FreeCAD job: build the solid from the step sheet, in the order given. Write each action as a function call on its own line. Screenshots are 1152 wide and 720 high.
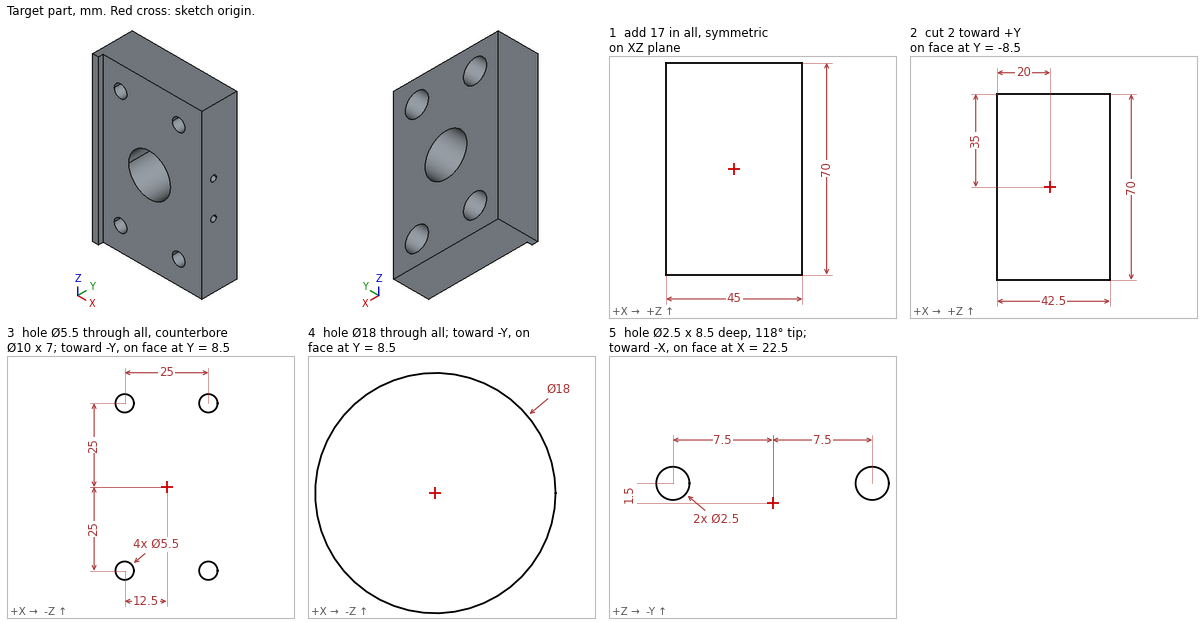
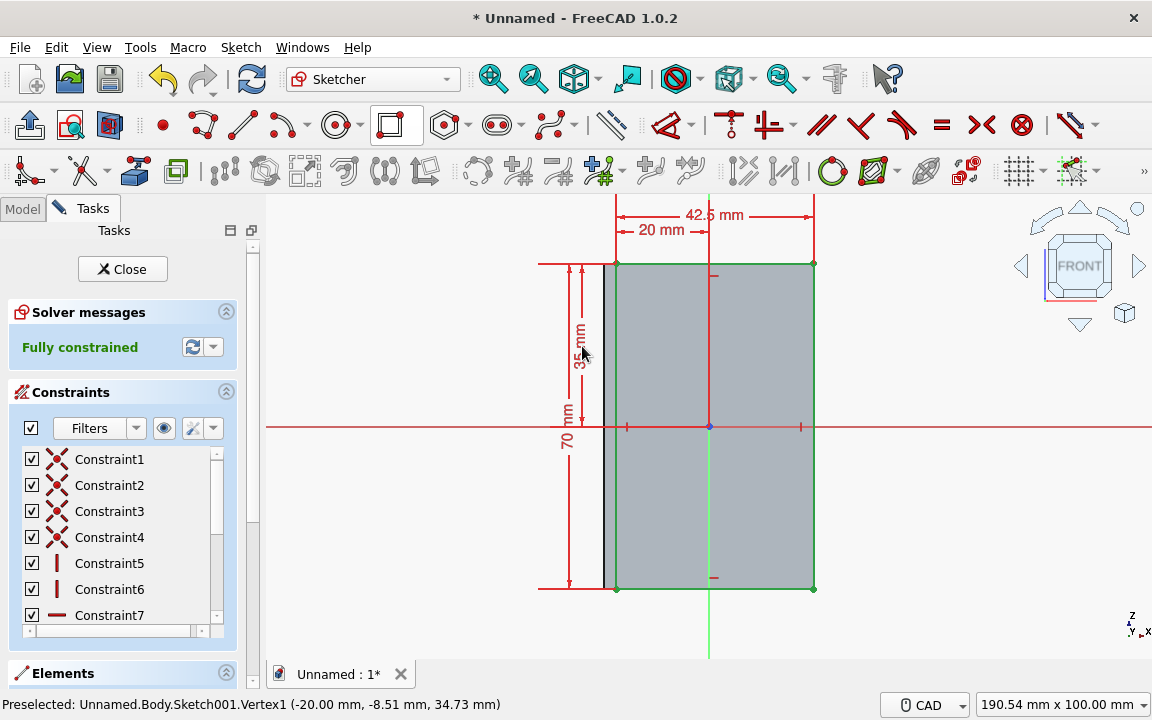
click(123, 269)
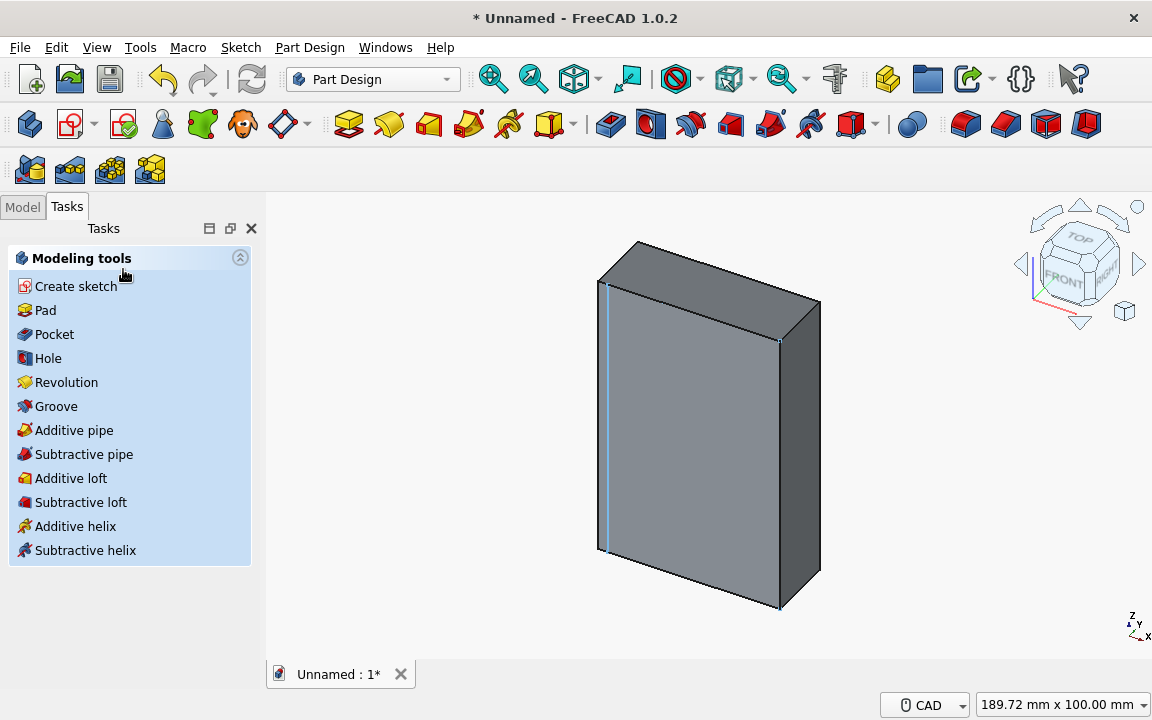
click(612, 124)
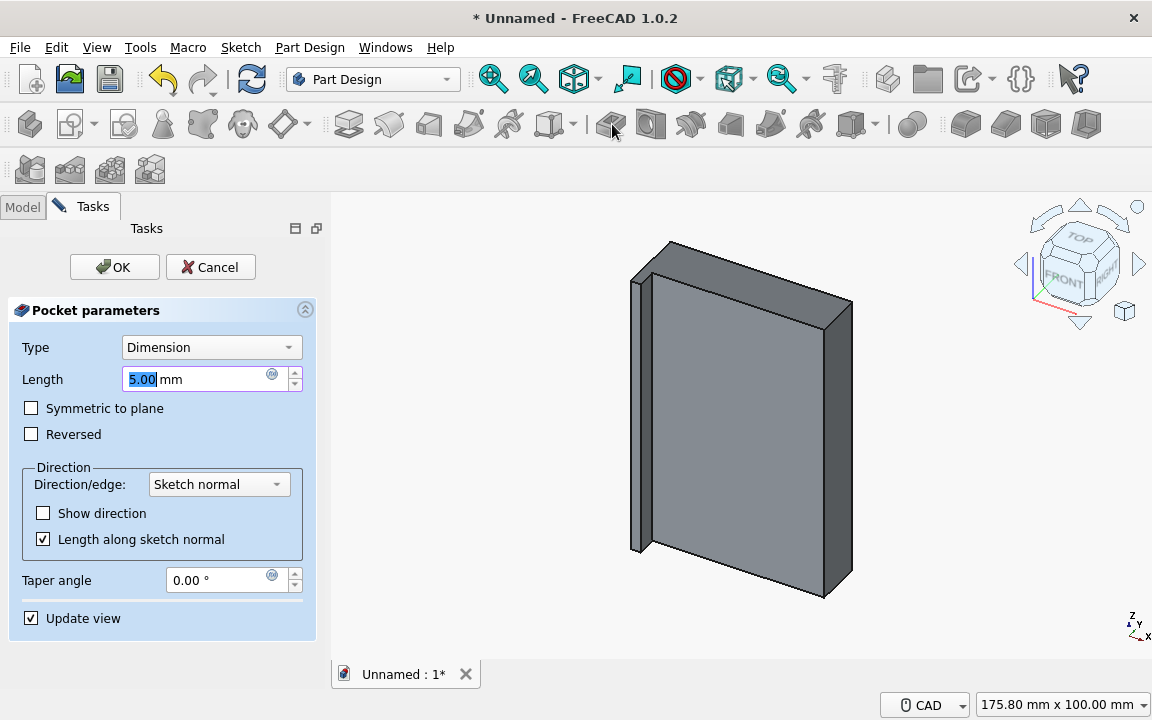
text(2)
key(Tab)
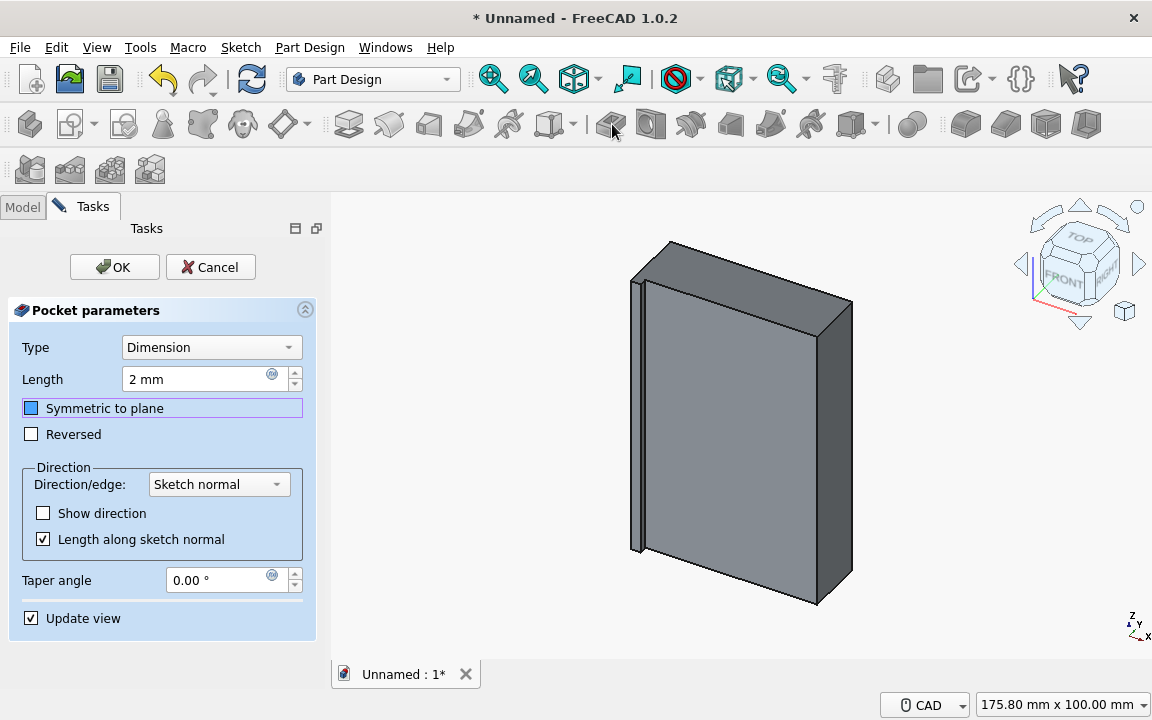
click(115, 267)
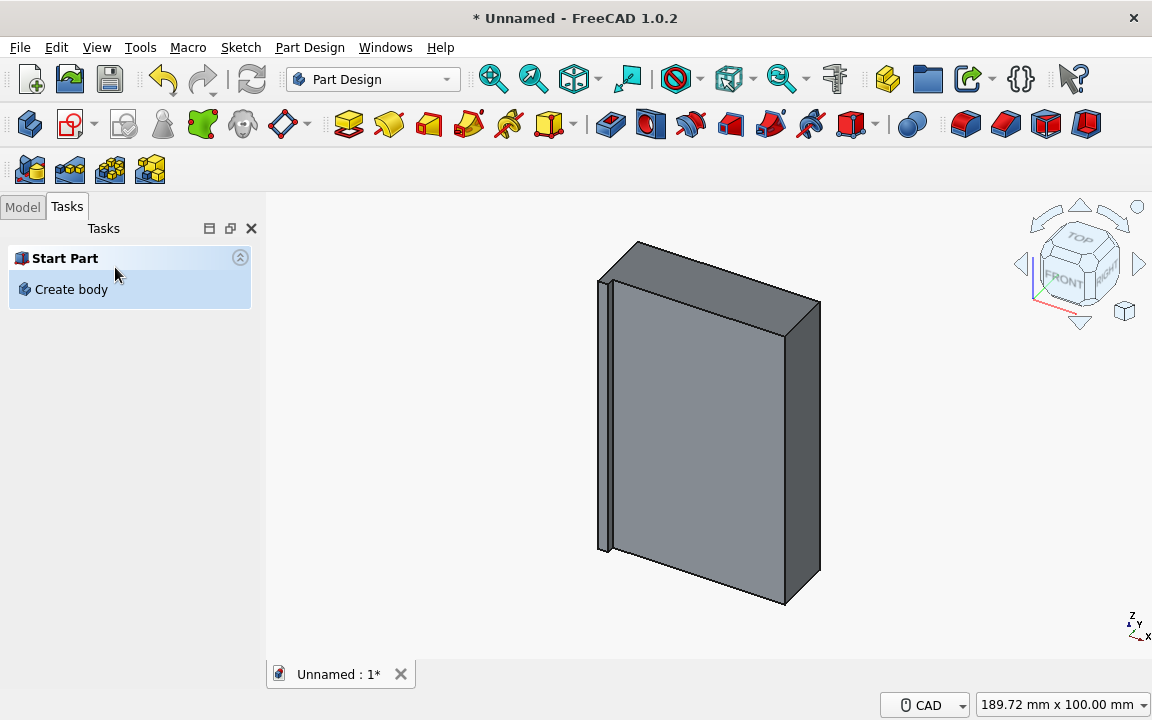
key(4)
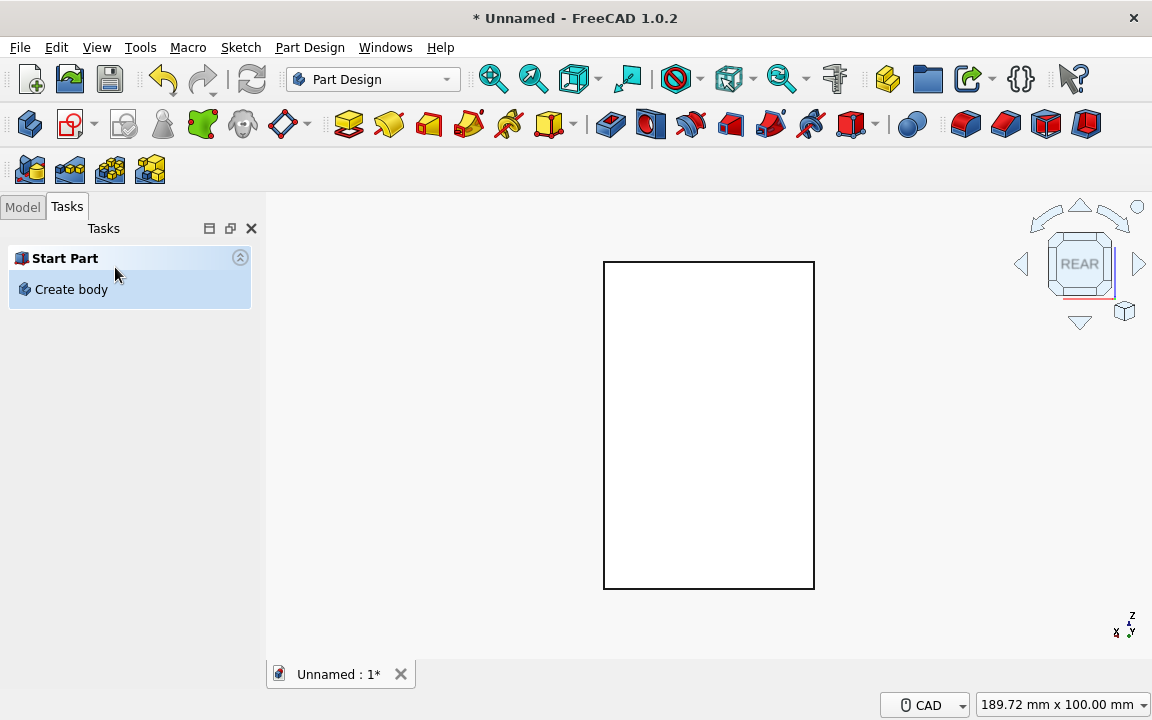
click(709, 378)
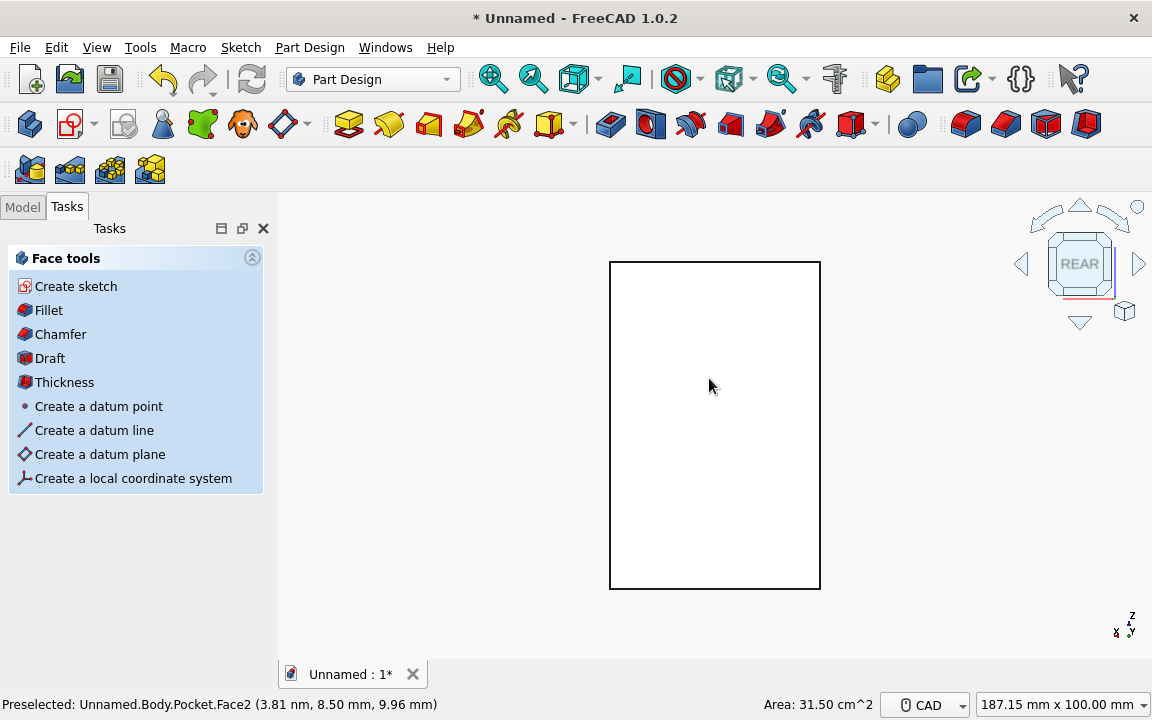
click(70, 124)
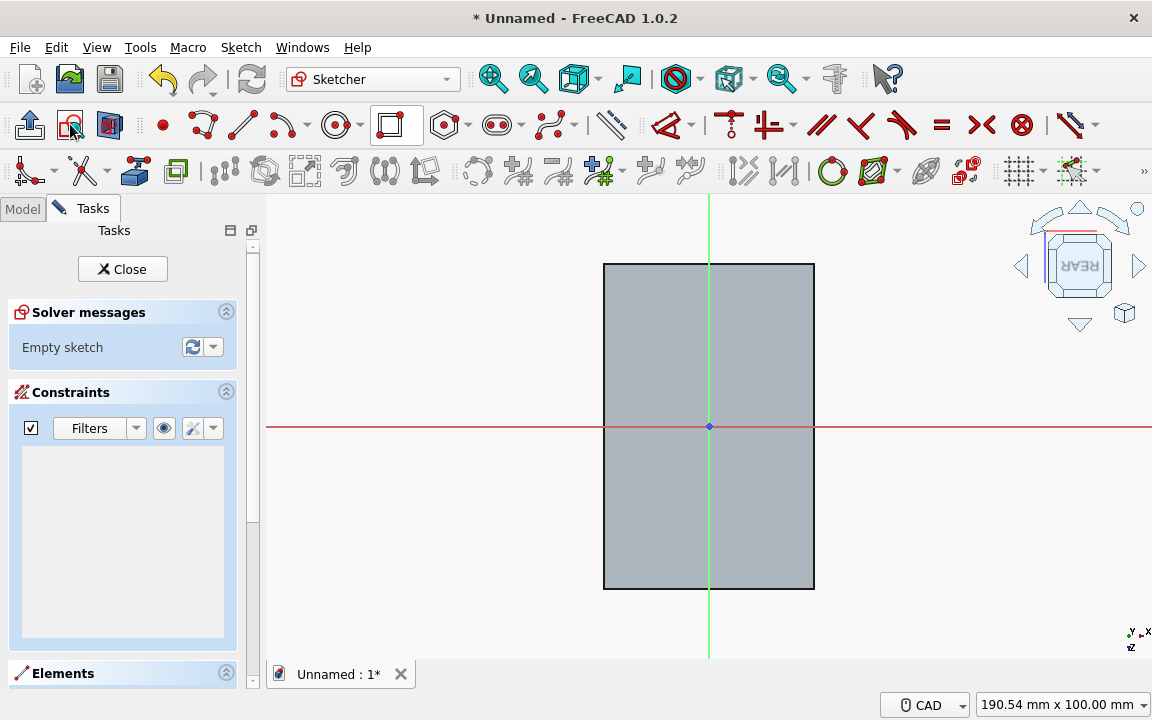
click(336, 126)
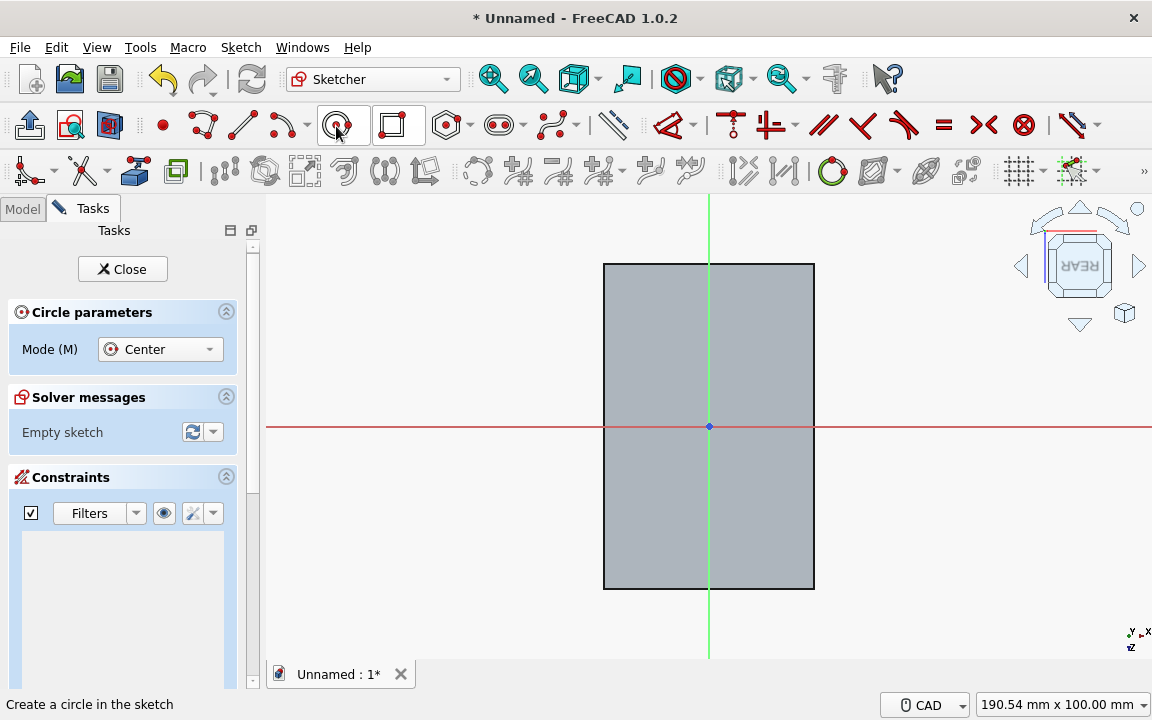
scroll(651, 543, up, 3)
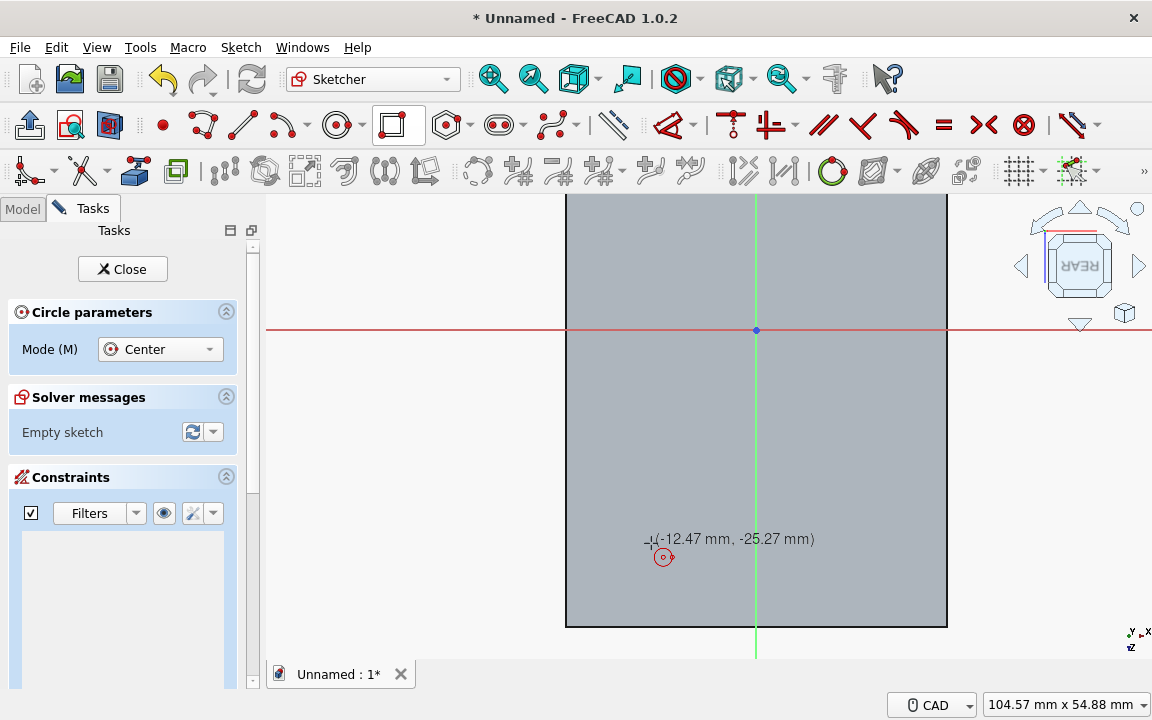
click(650, 542)
move(667, 525)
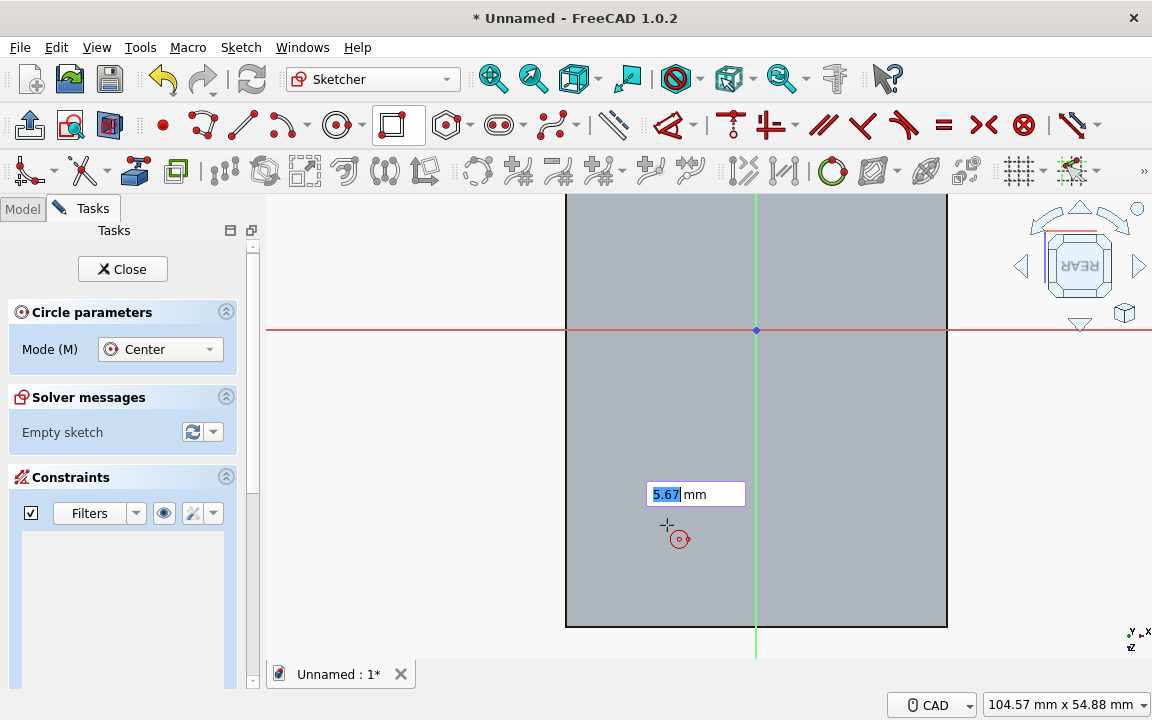
text(5.5)
key(Return)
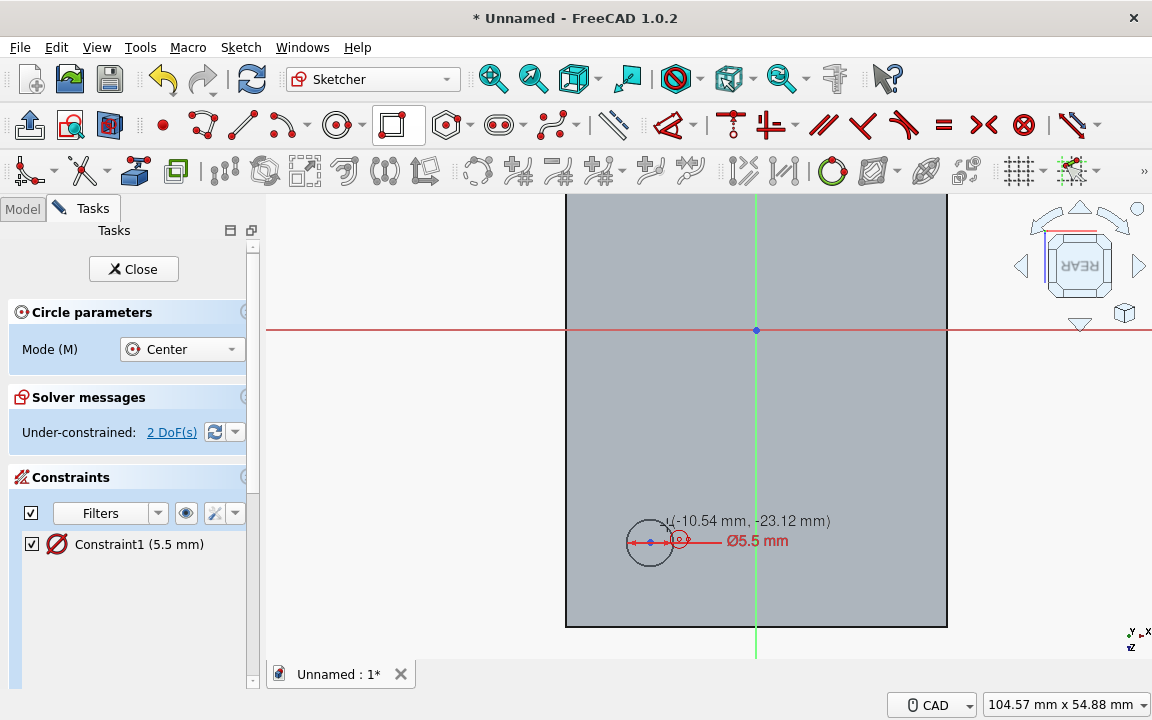
scroll(405, 622, down, 2)